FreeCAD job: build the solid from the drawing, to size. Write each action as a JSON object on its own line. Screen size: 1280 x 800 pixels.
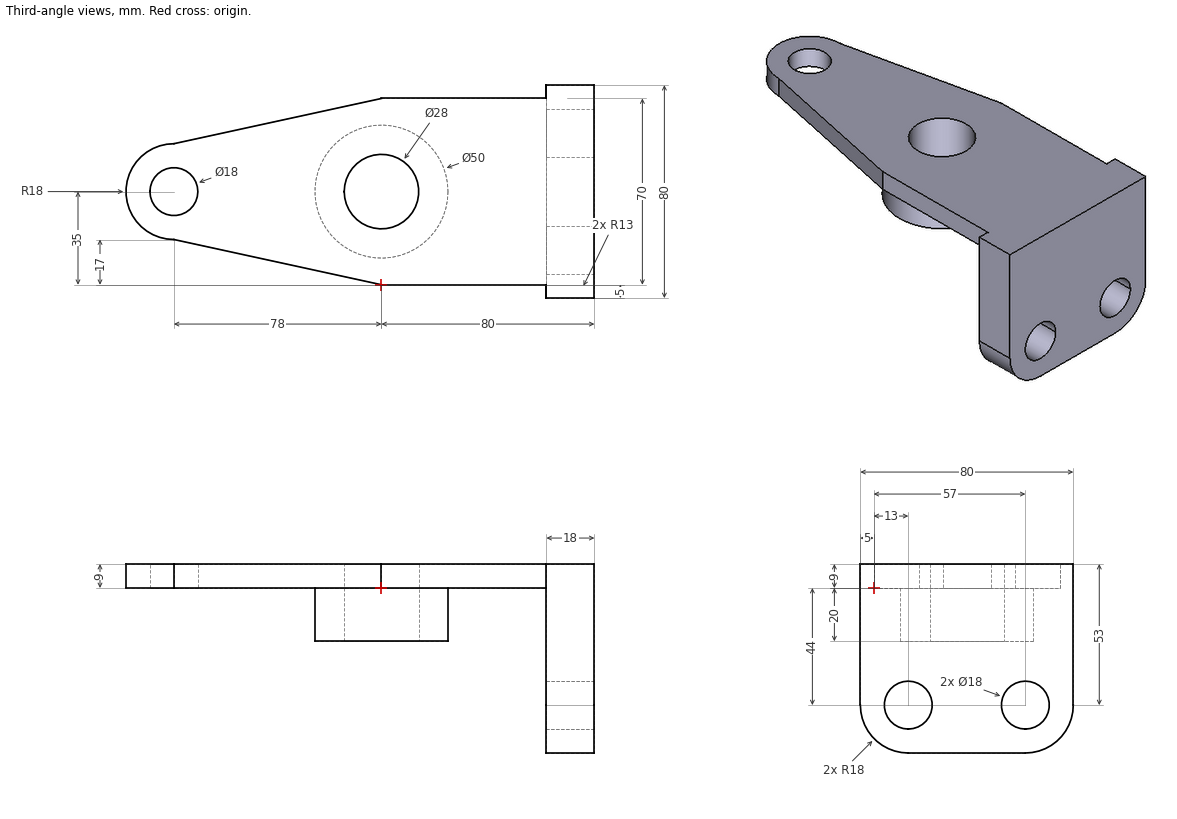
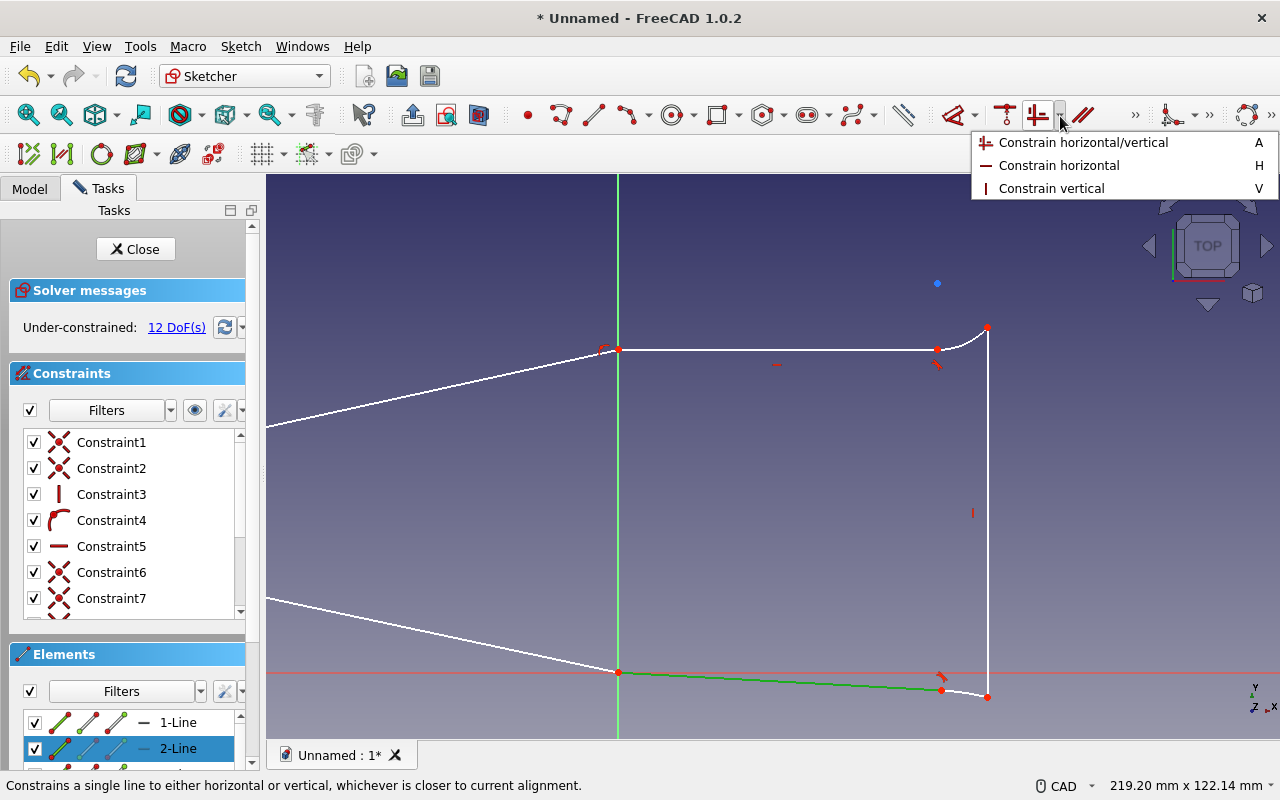
{"action": "left_click", "coordinate": [1125, 166]}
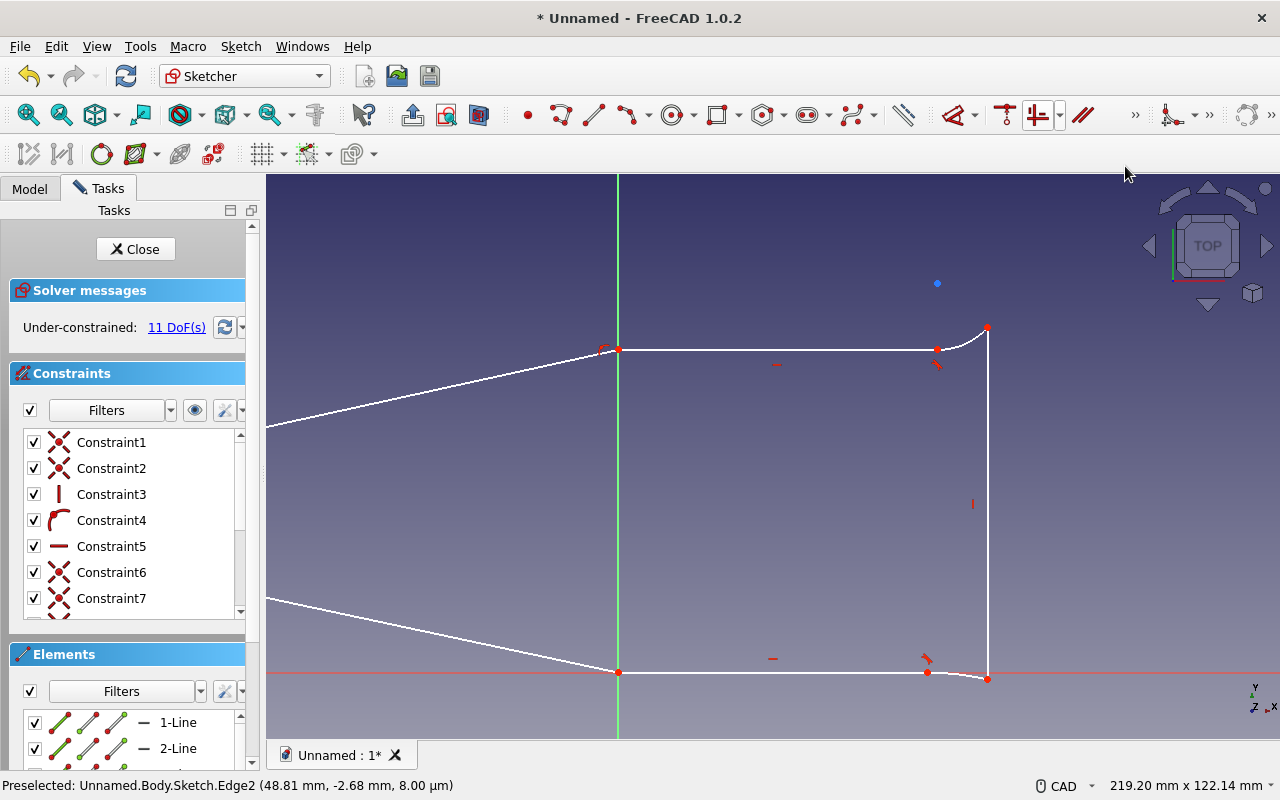
{"action": "left_click", "coordinate": [970, 676]}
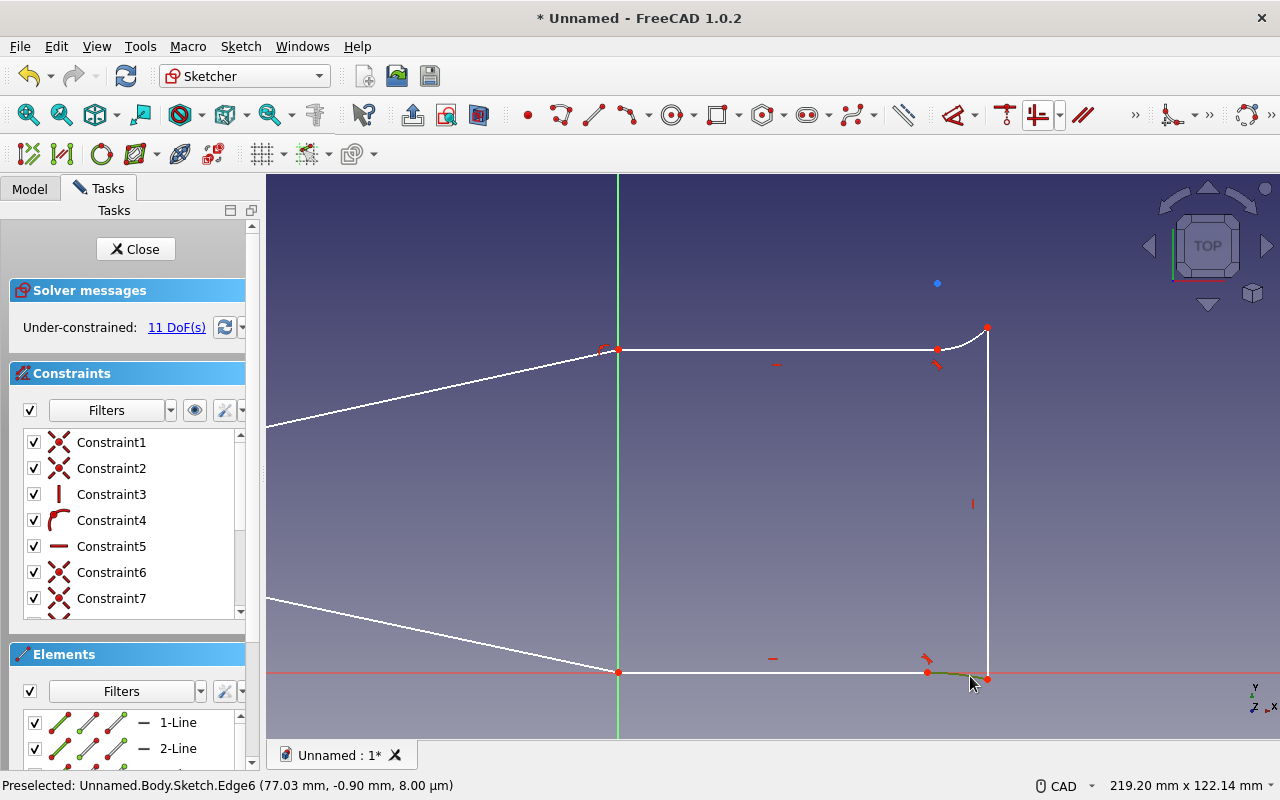
{"action": "left_click", "coordinate": [954, 348]}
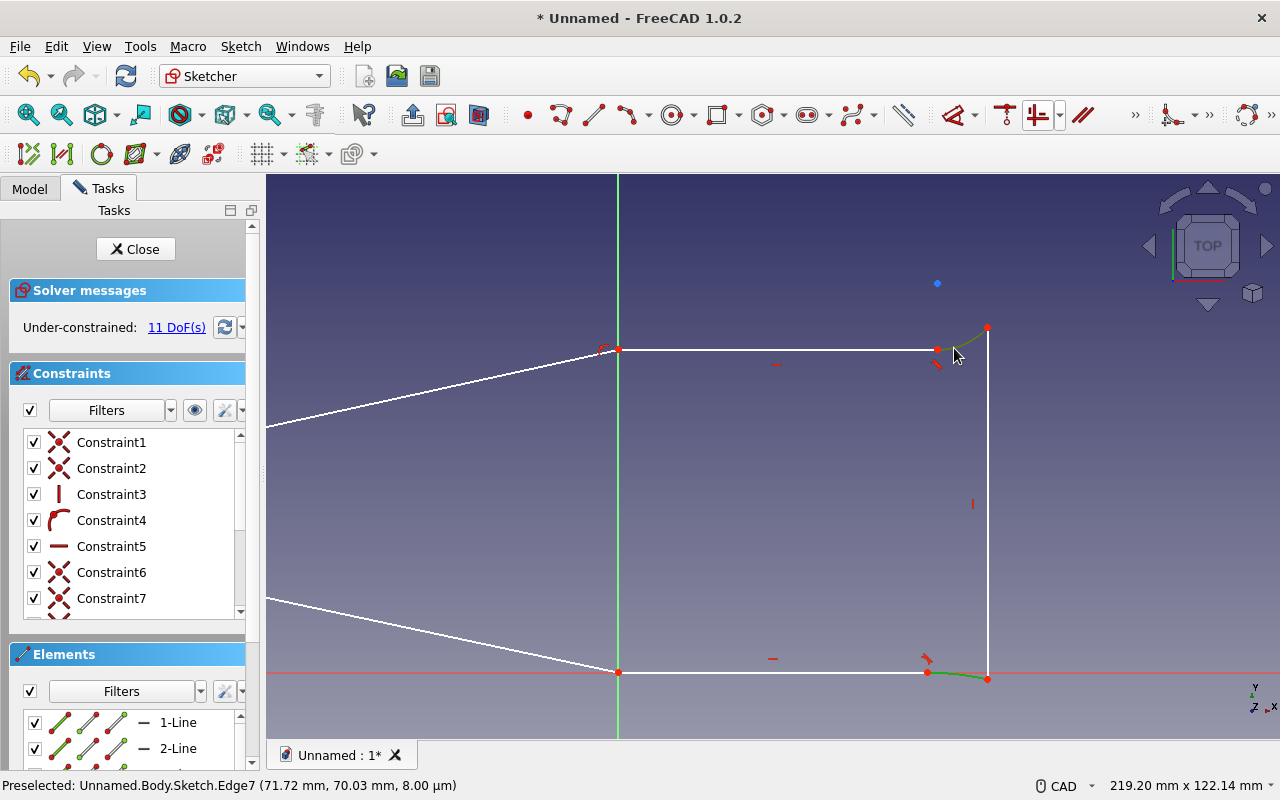
{"action": "key", "text": "e"}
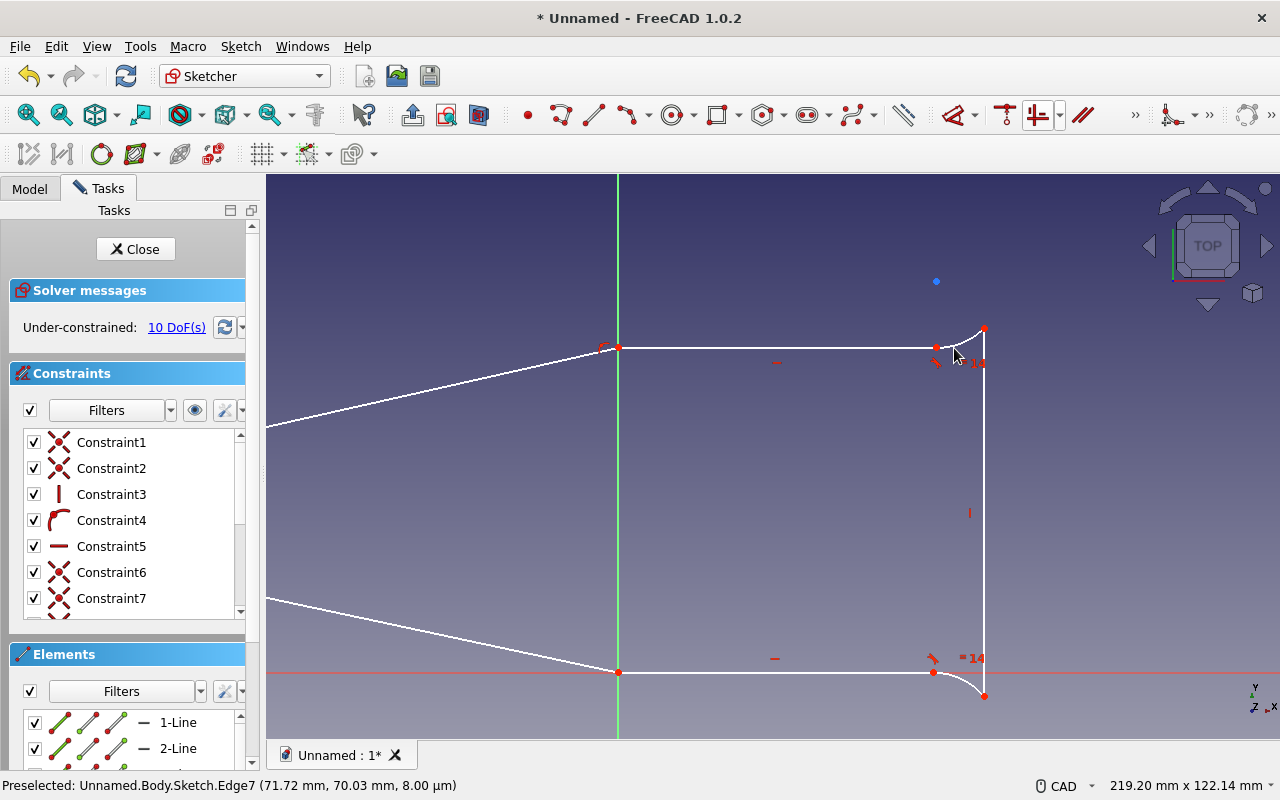
{"action": "left_click", "coordinate": [952, 116]}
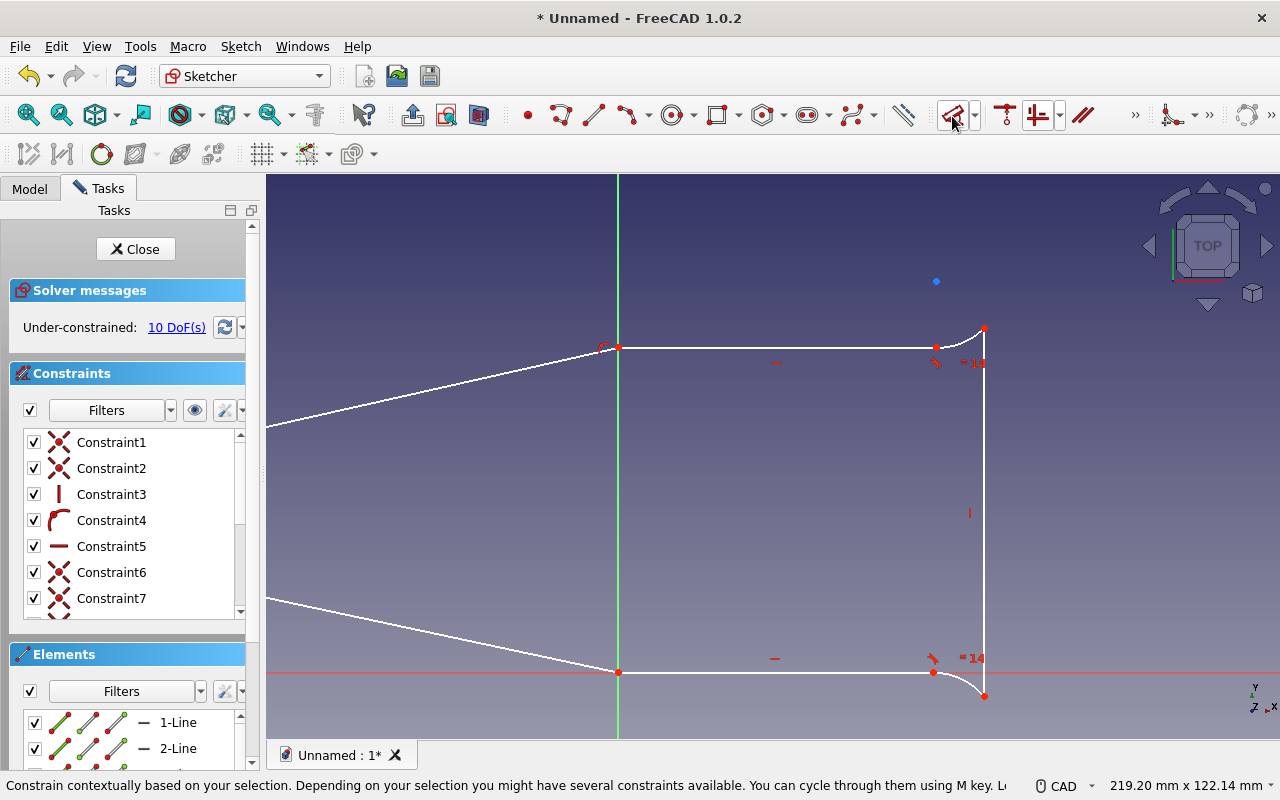
{"action": "left_click", "coordinate": [971, 685]}
{"action": "left_click", "coordinate": [1021, 696]}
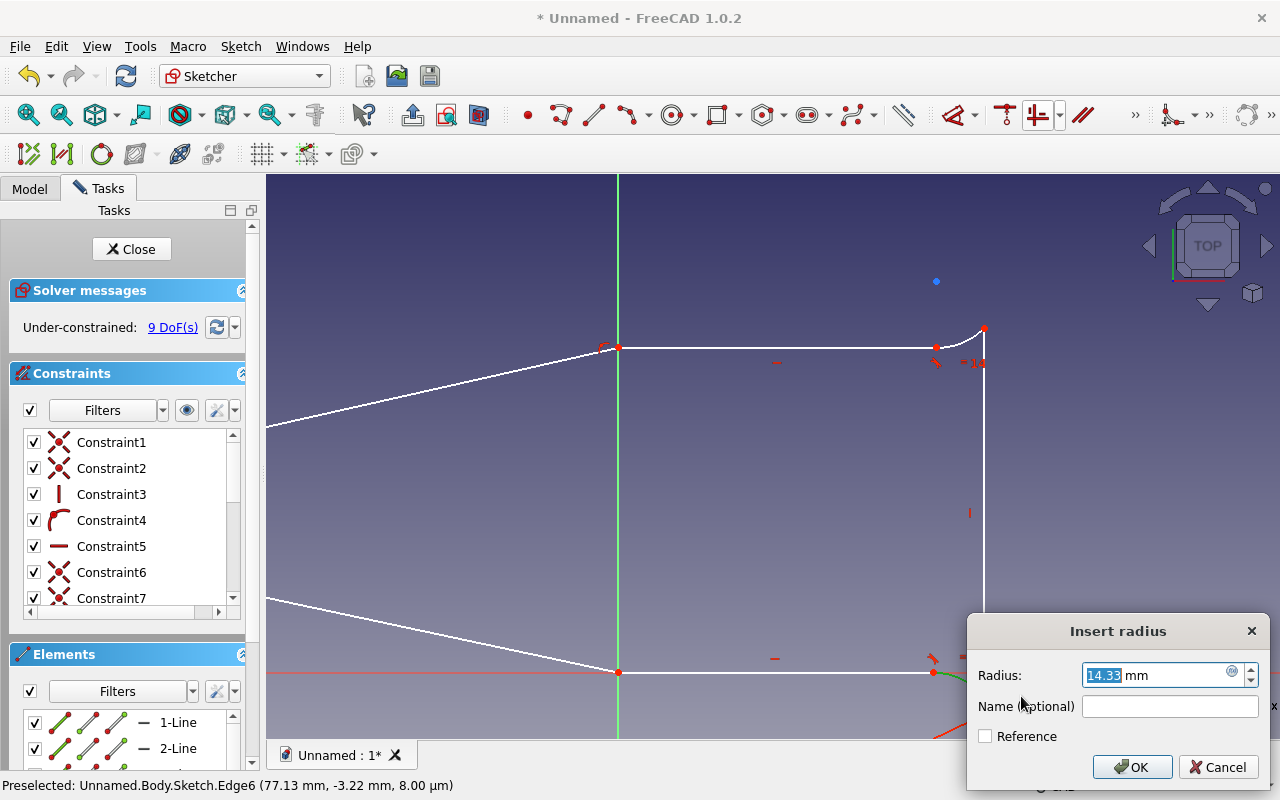
{"action": "type", "text": "13"}
{"action": "key", "text": "Return"}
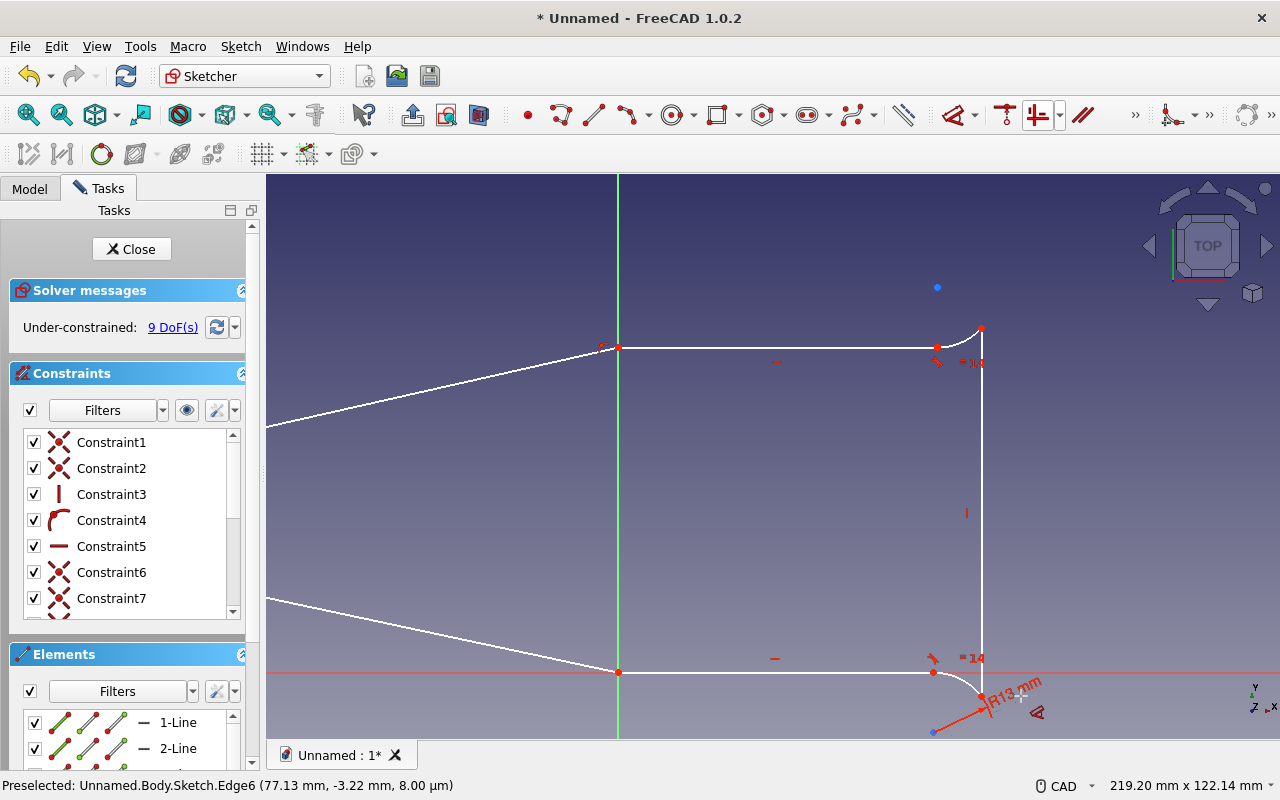
{"action": "scroll", "coordinate": [955, 346], "scroll_direction": "down", "scroll_amount": 2}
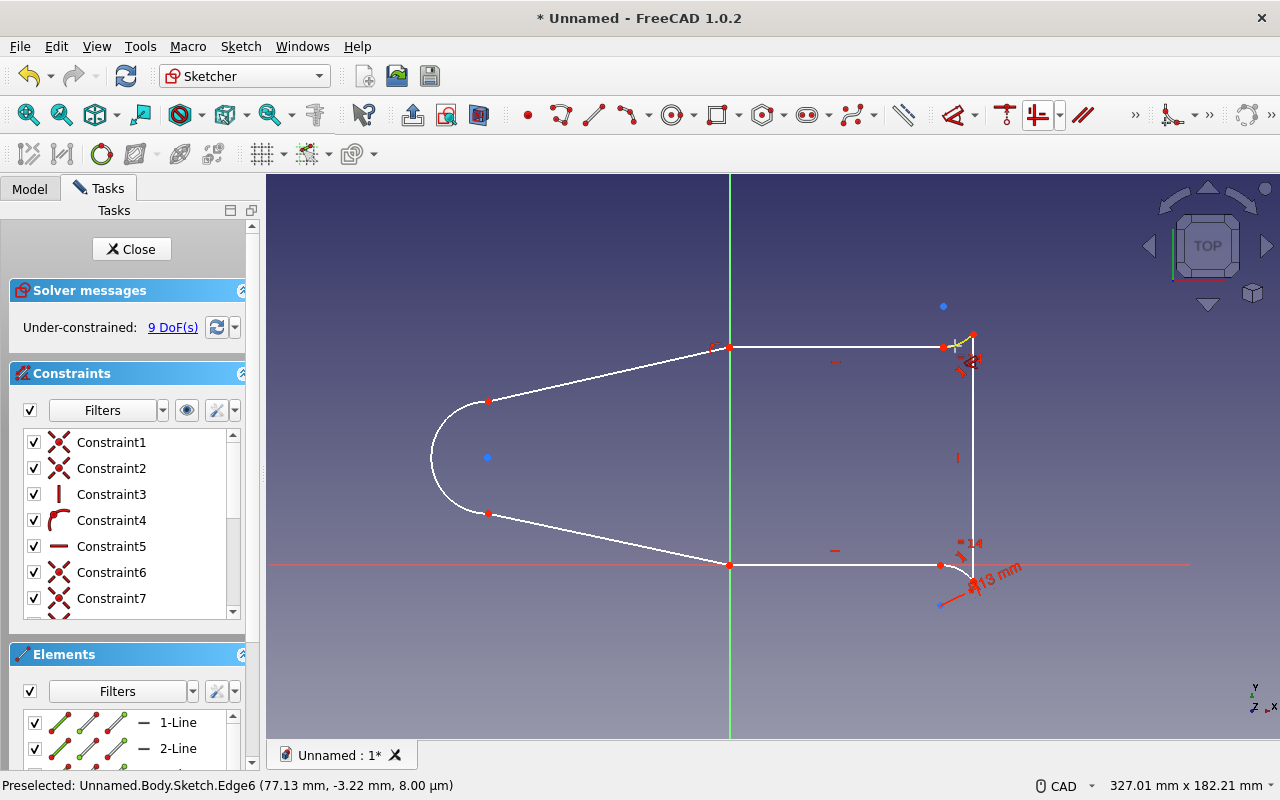
{"action": "left_click", "coordinate": [442, 425]}
{"action": "left_click", "coordinate": [416, 406]}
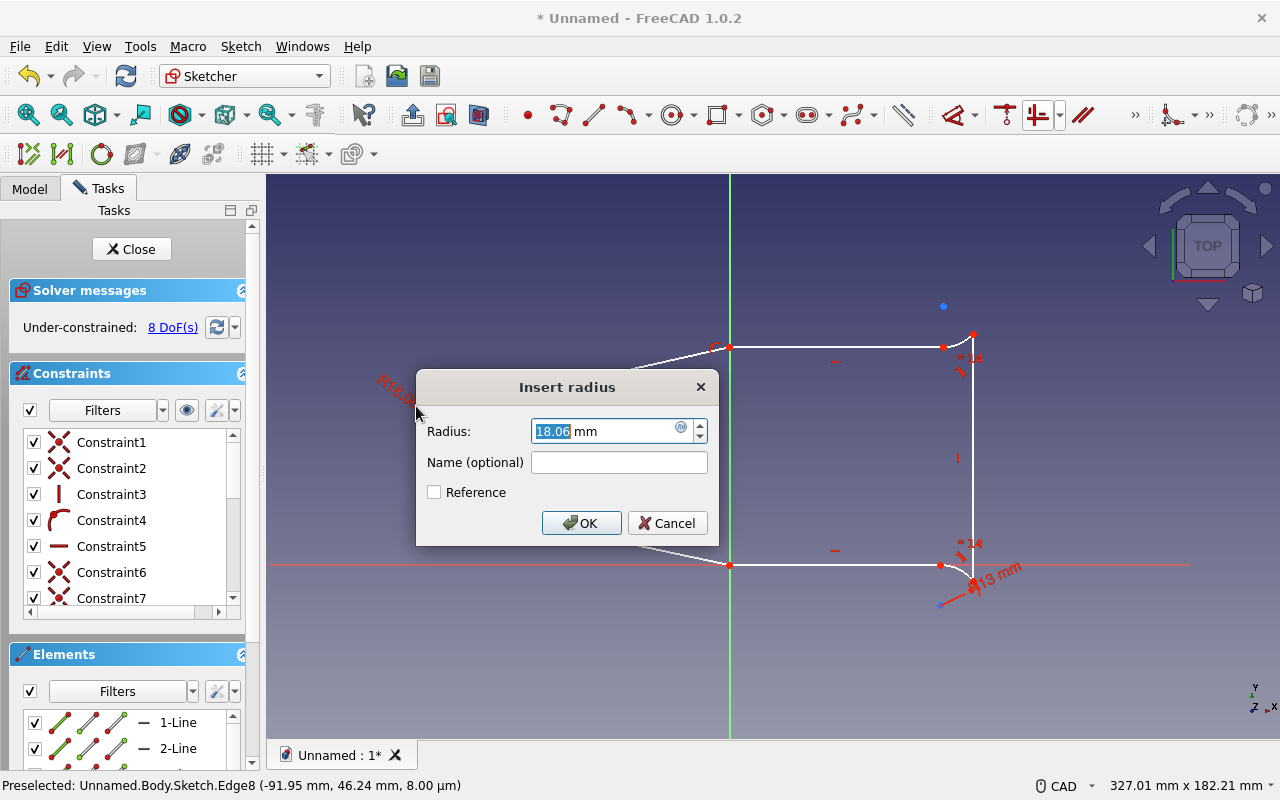
{"action": "type", "text": "18"}
{"action": "key", "text": "Return"}